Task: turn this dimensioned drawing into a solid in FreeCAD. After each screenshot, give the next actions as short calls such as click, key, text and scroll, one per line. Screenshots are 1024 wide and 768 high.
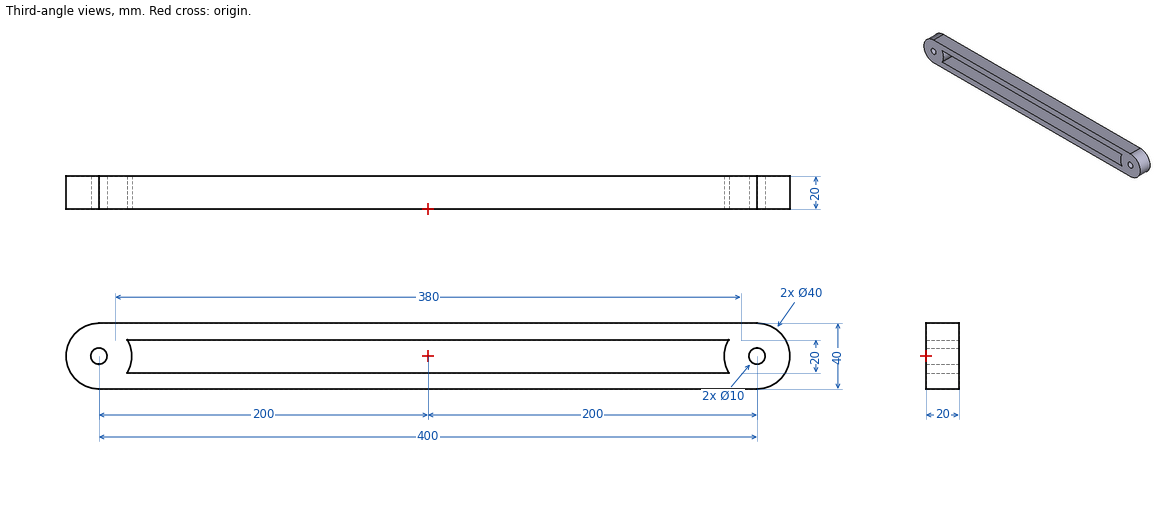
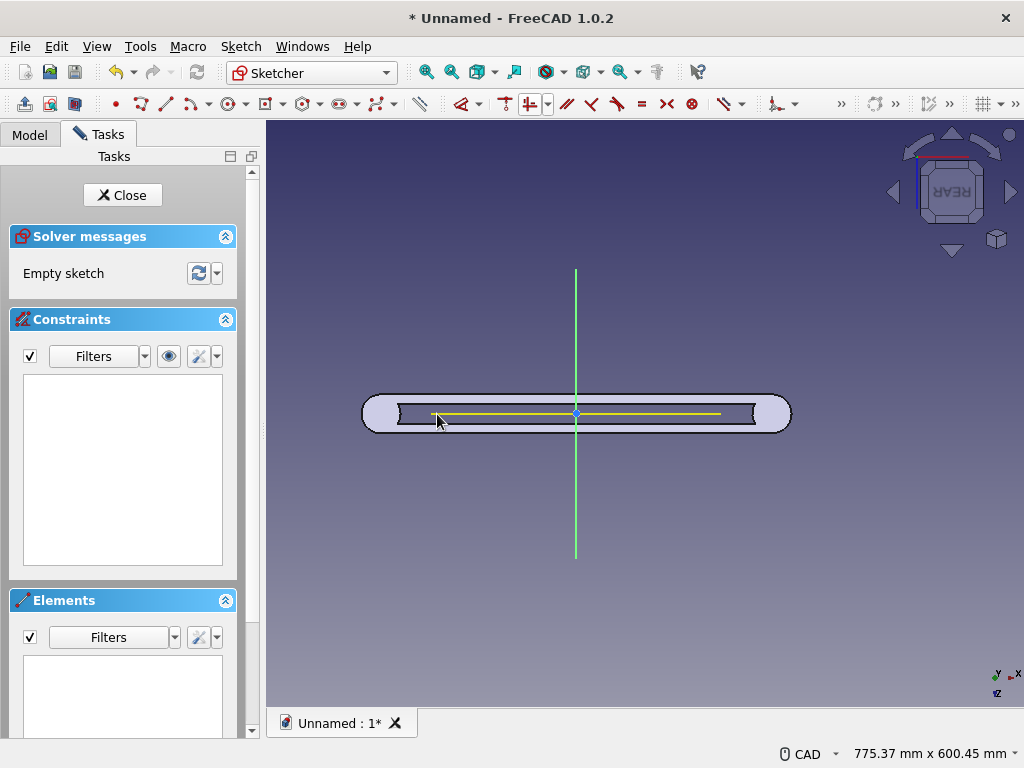
click(228, 104)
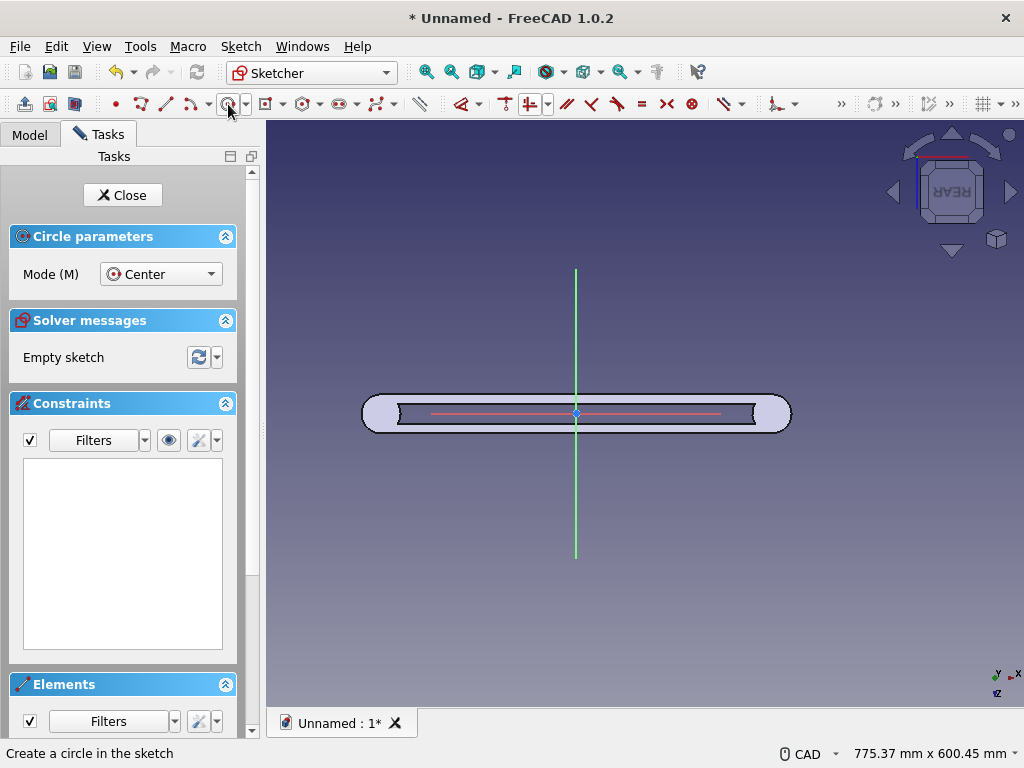
scroll(772, 414, up, 8)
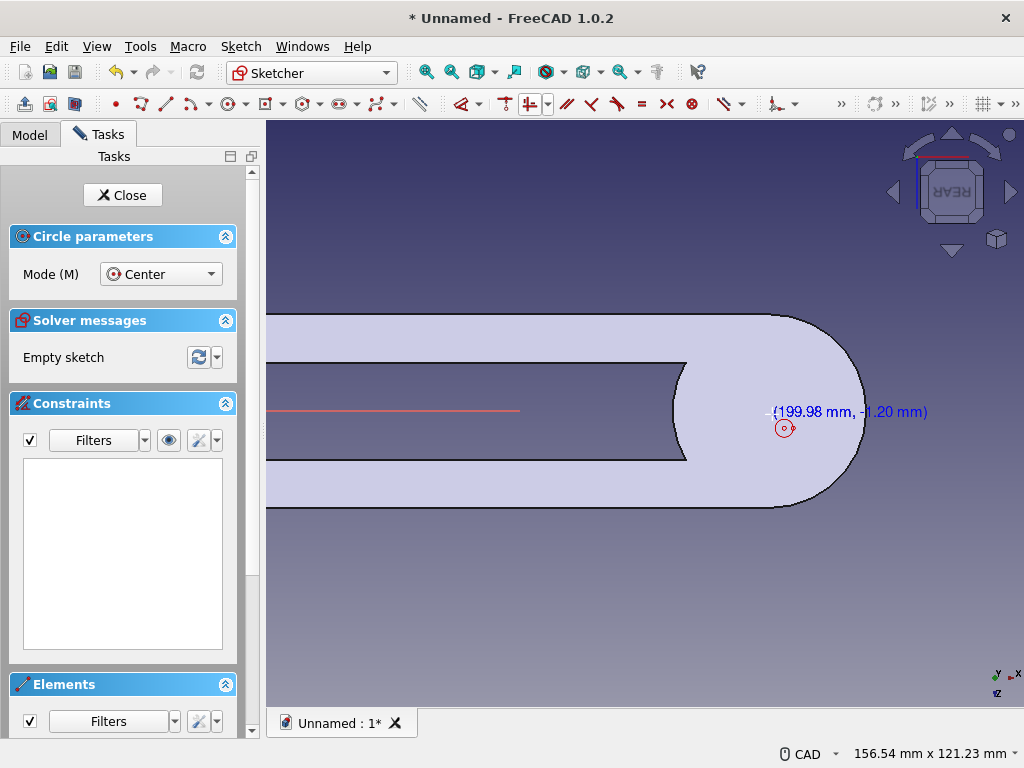
scroll(773, 414, down, 8)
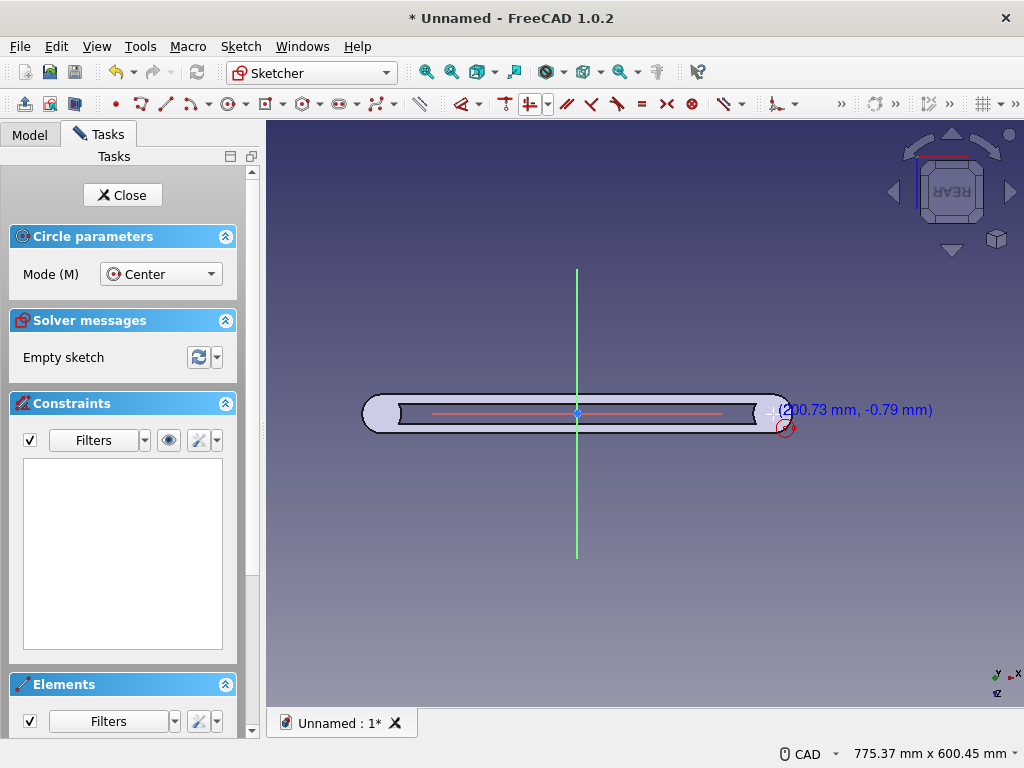
click(773, 414)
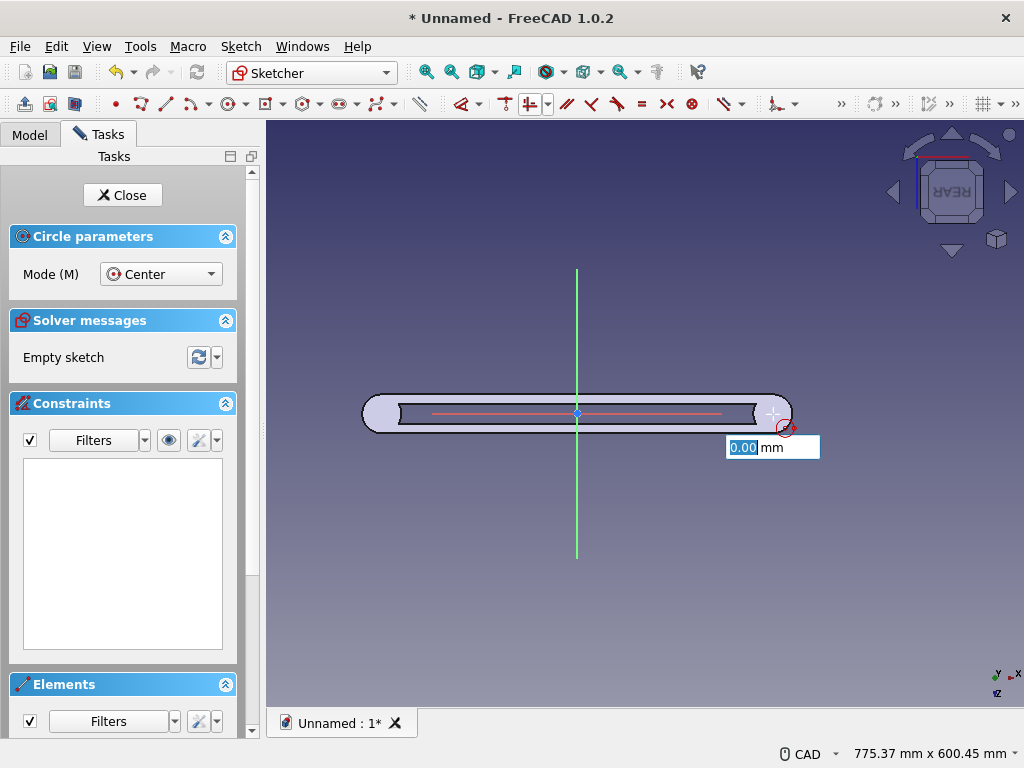
scroll(774, 409, up, 7)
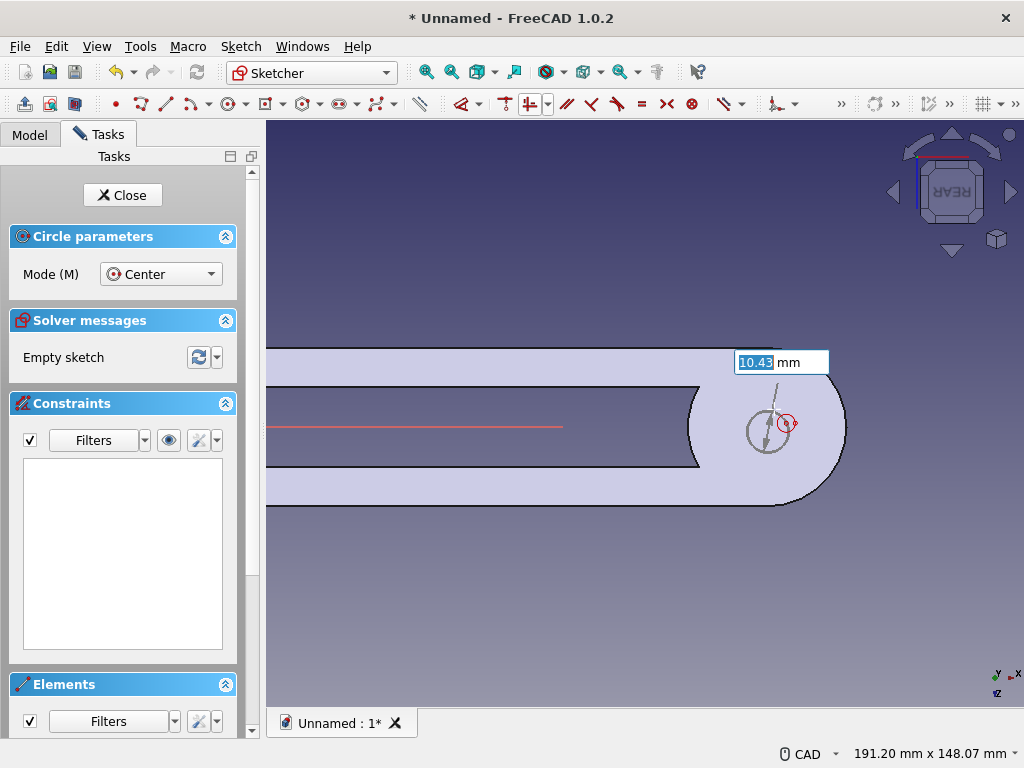
click(774, 408)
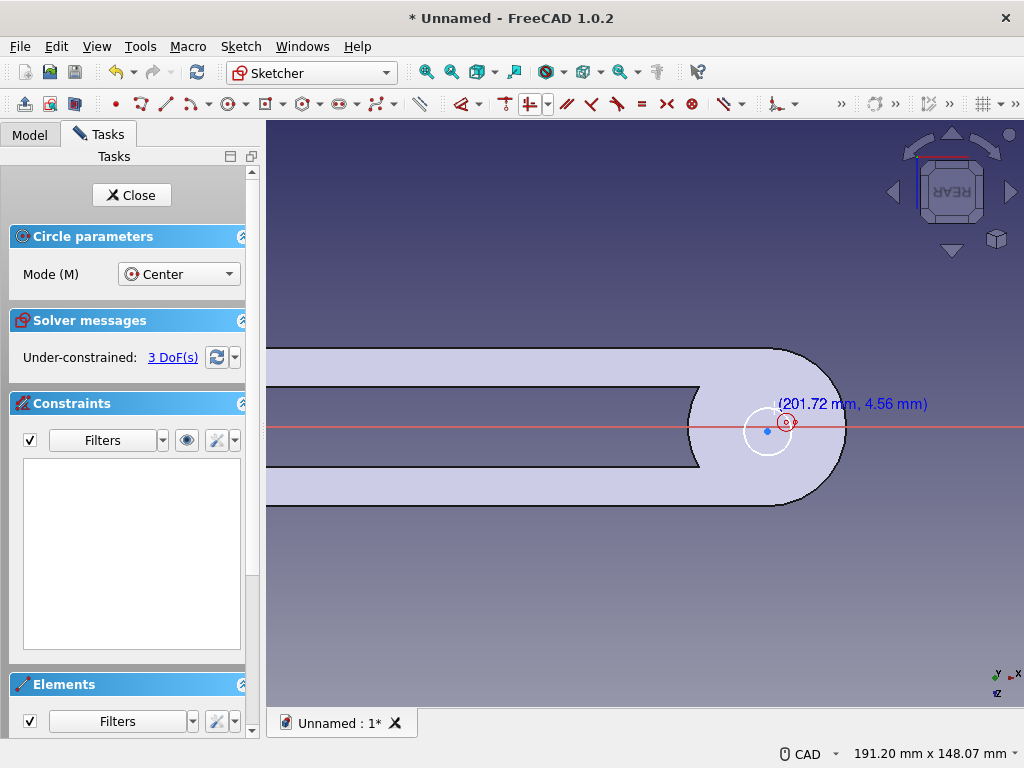
scroll(774, 409, down, 7)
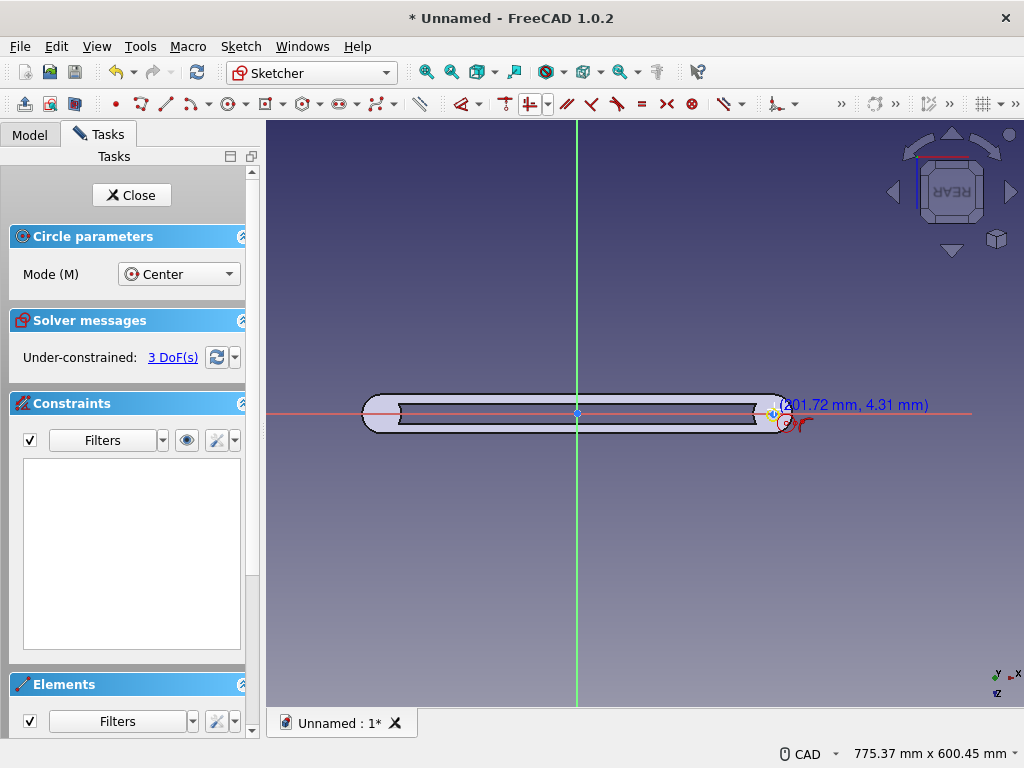
scroll(382, 414, up, 8)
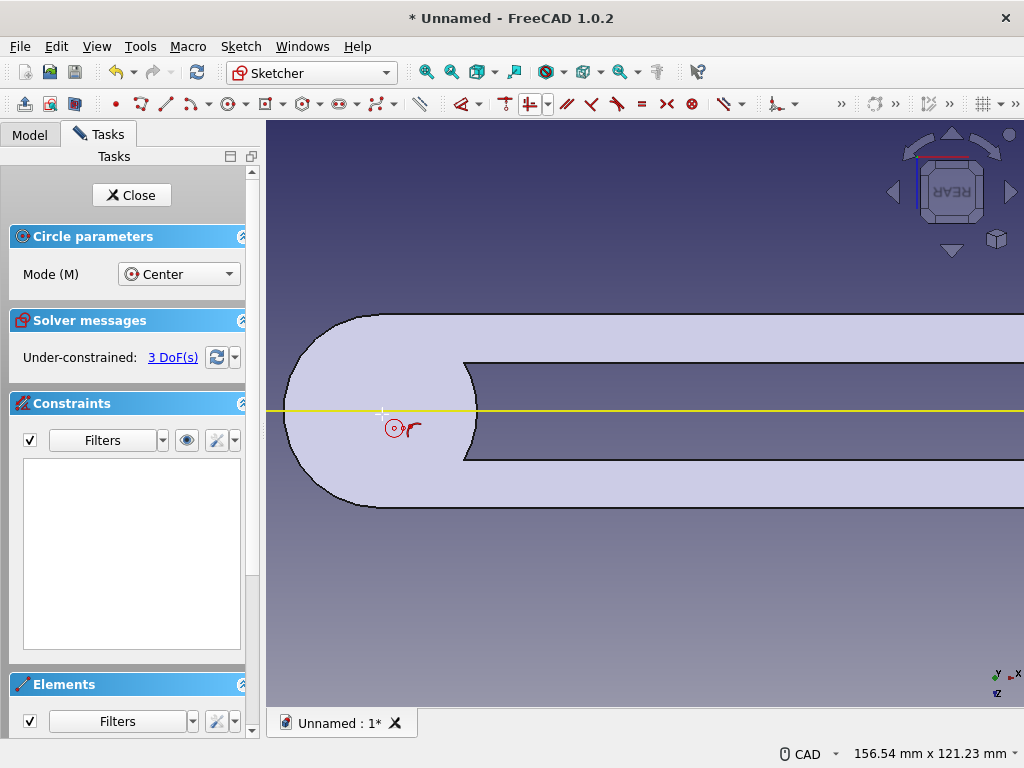
scroll(381, 414, down, 8)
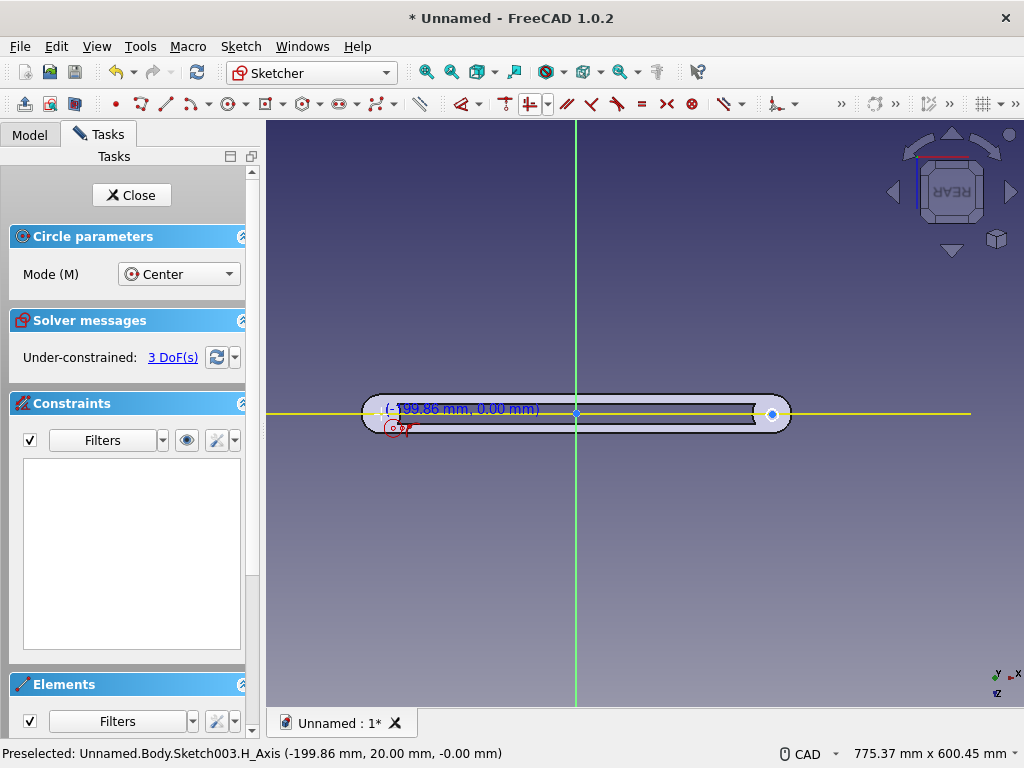
click(381, 414)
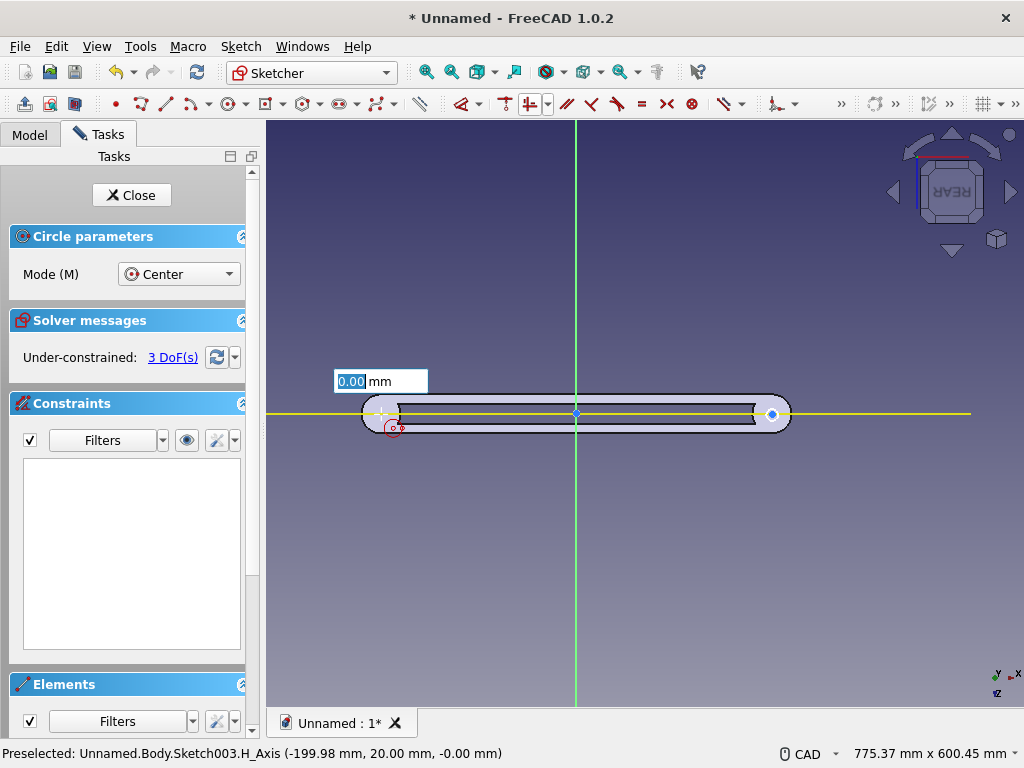
scroll(379, 418, up, 7)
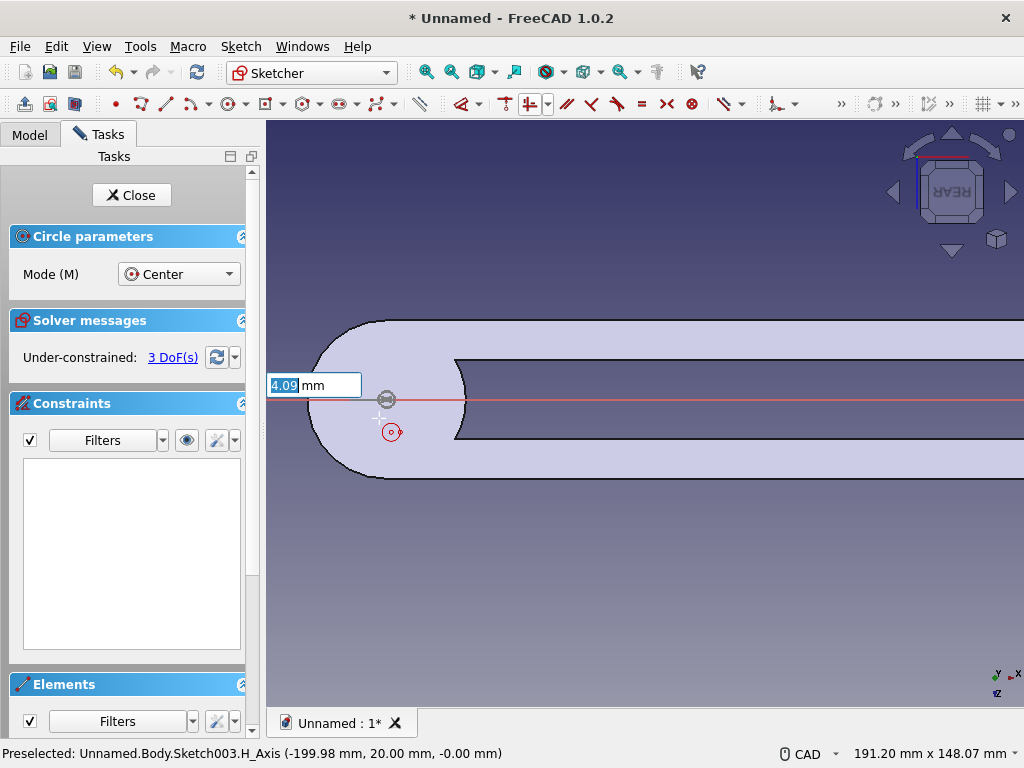
click(380, 418)
key(Escape)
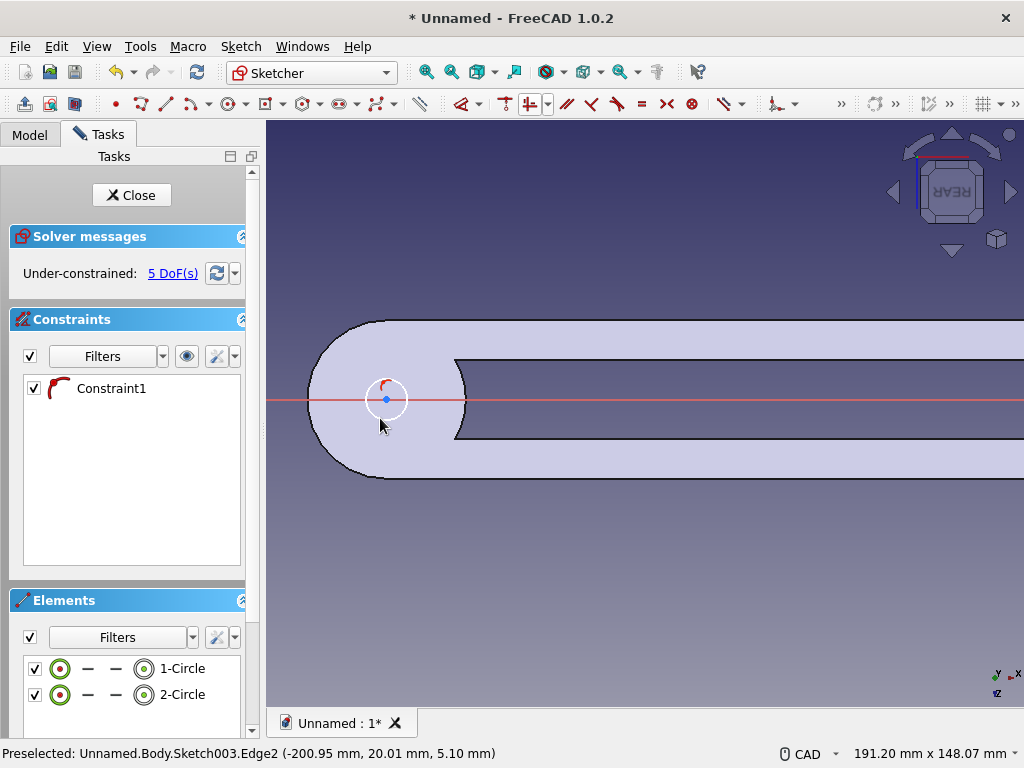
scroll(379, 418, down, 7)